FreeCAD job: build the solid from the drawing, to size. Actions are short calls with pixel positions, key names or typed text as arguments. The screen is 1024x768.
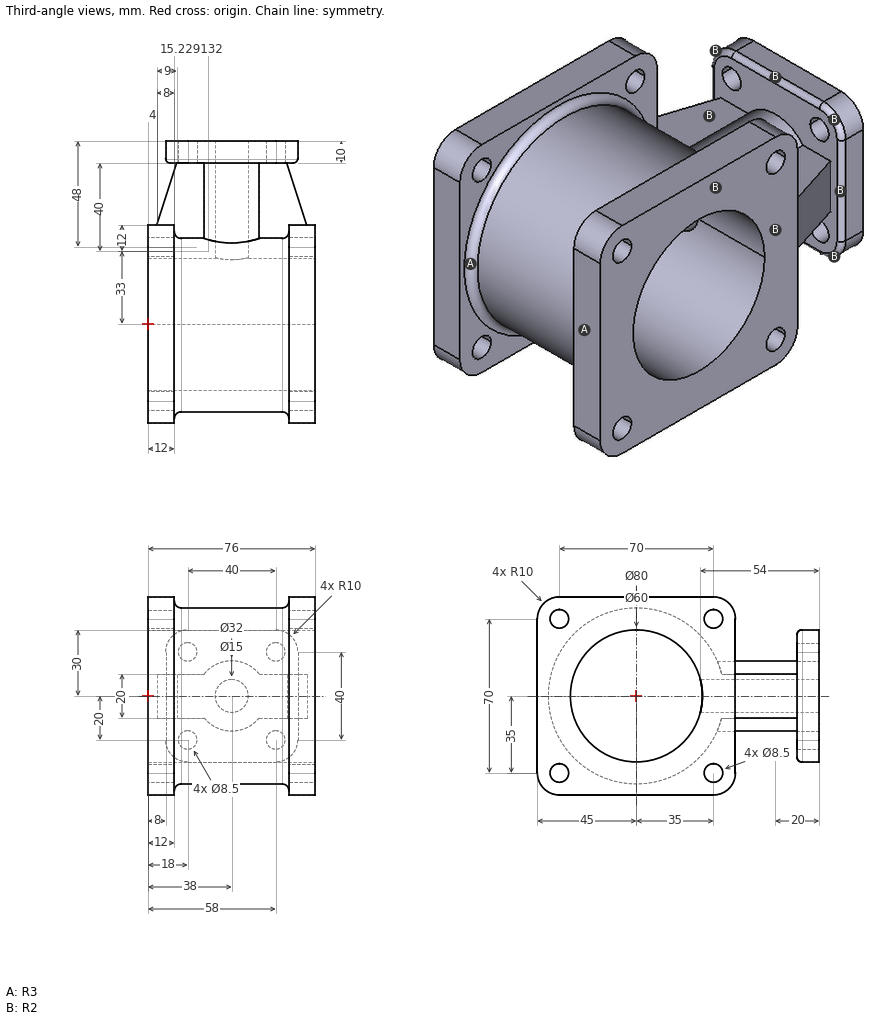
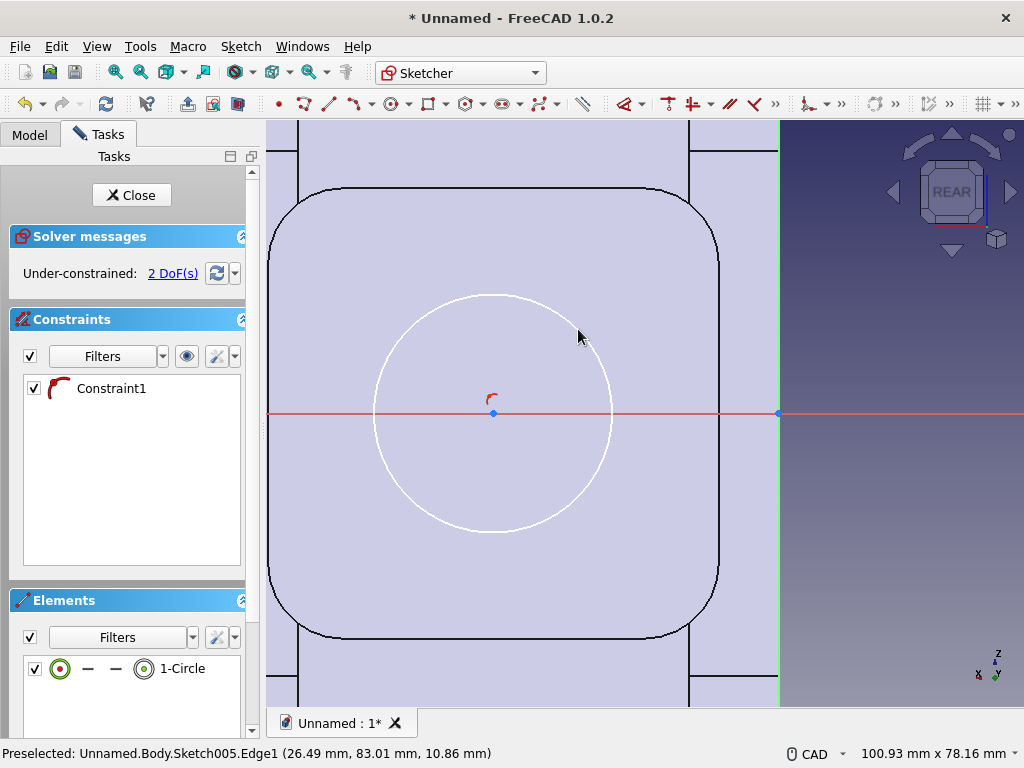
click(624, 104)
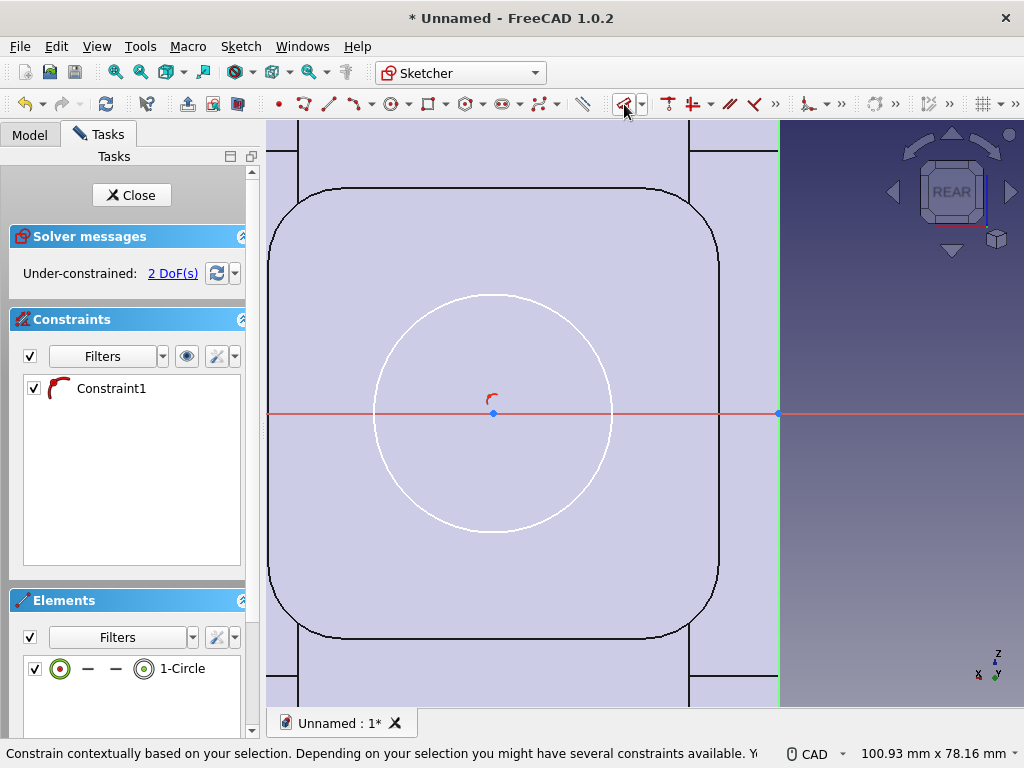
click(577, 329)
click(600, 306)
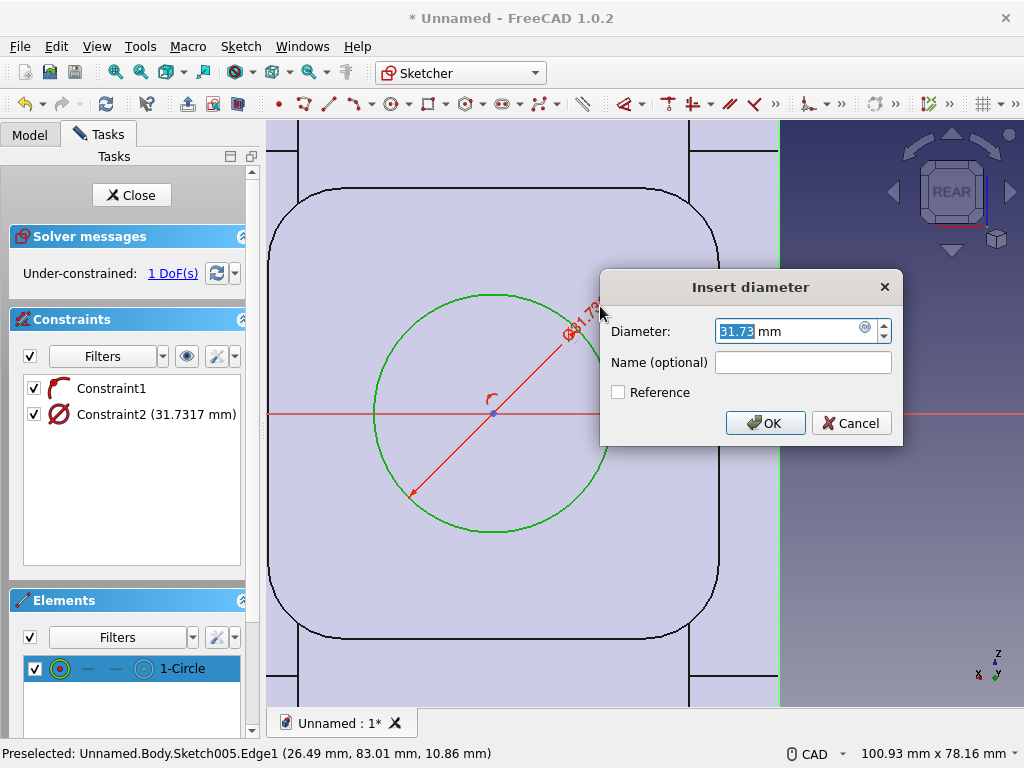
text(32)
key(Return)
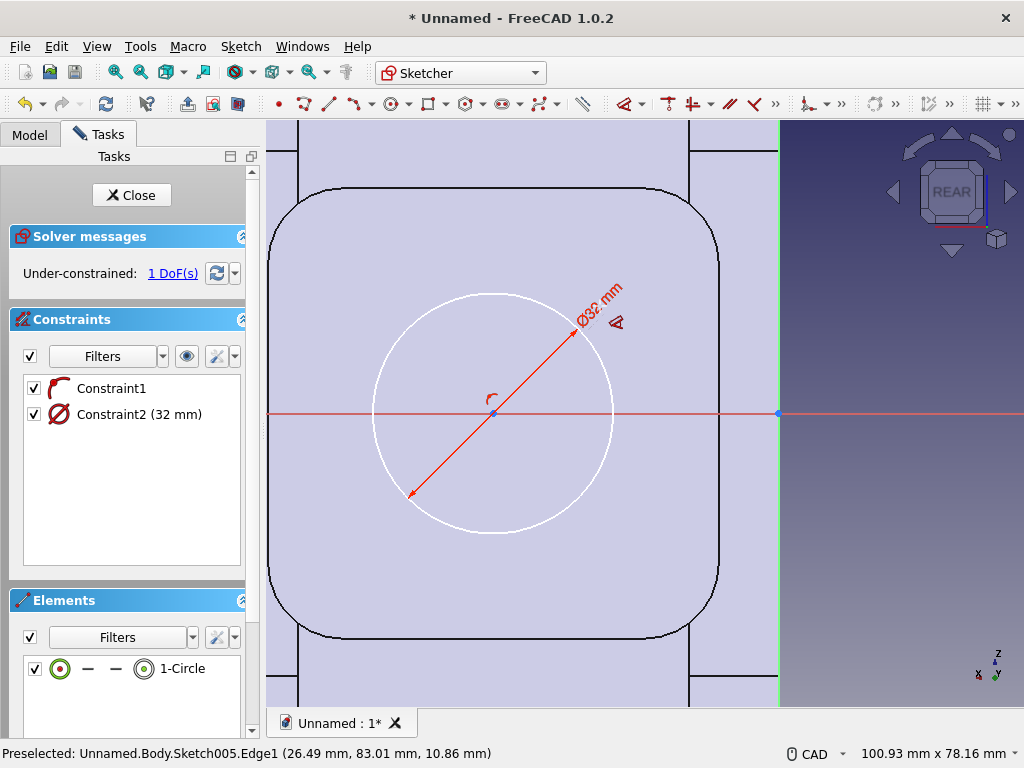
click(493, 413)
click(636, 447)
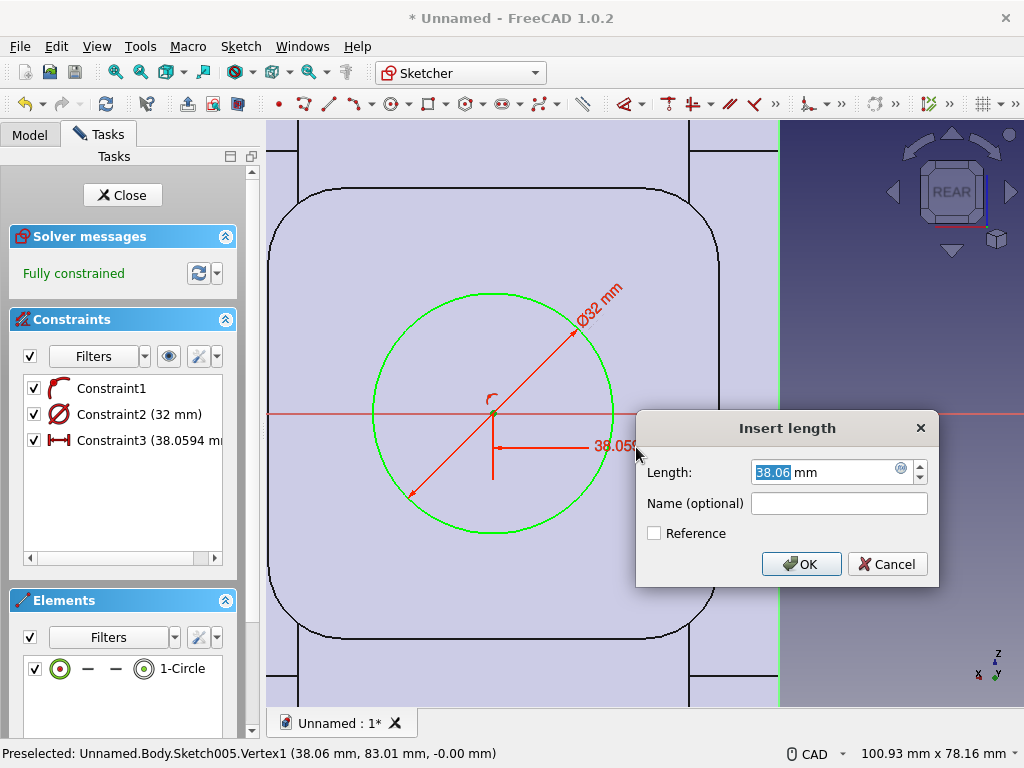
text(38)
key(Return)
key(Escape)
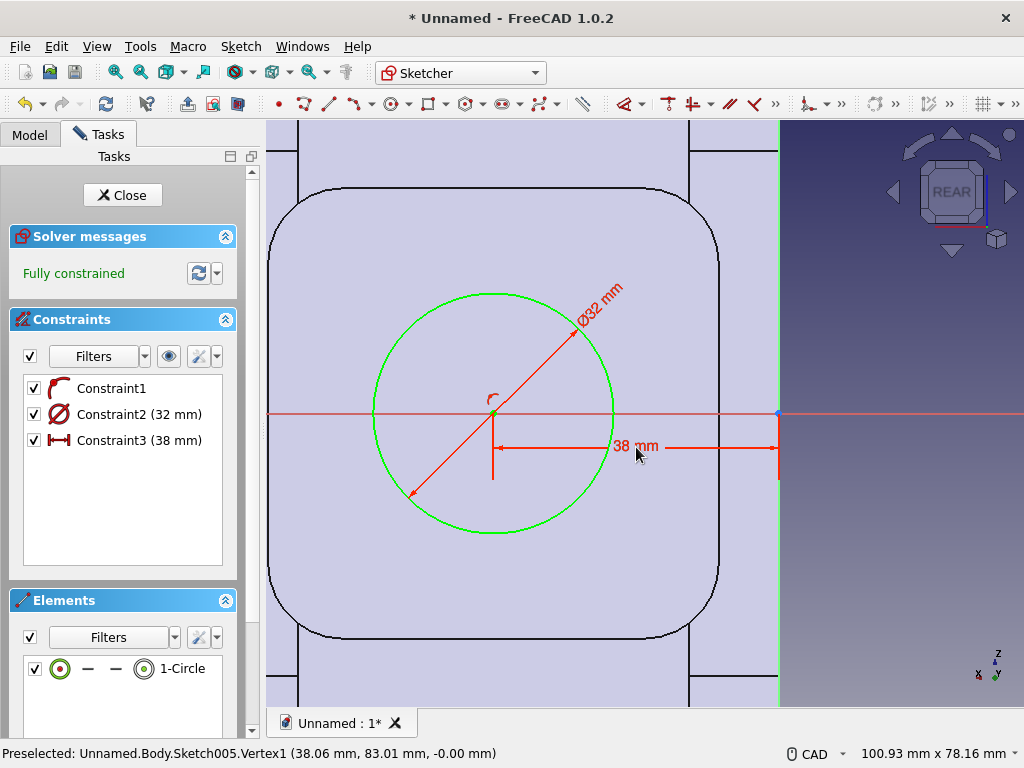
click(123, 195)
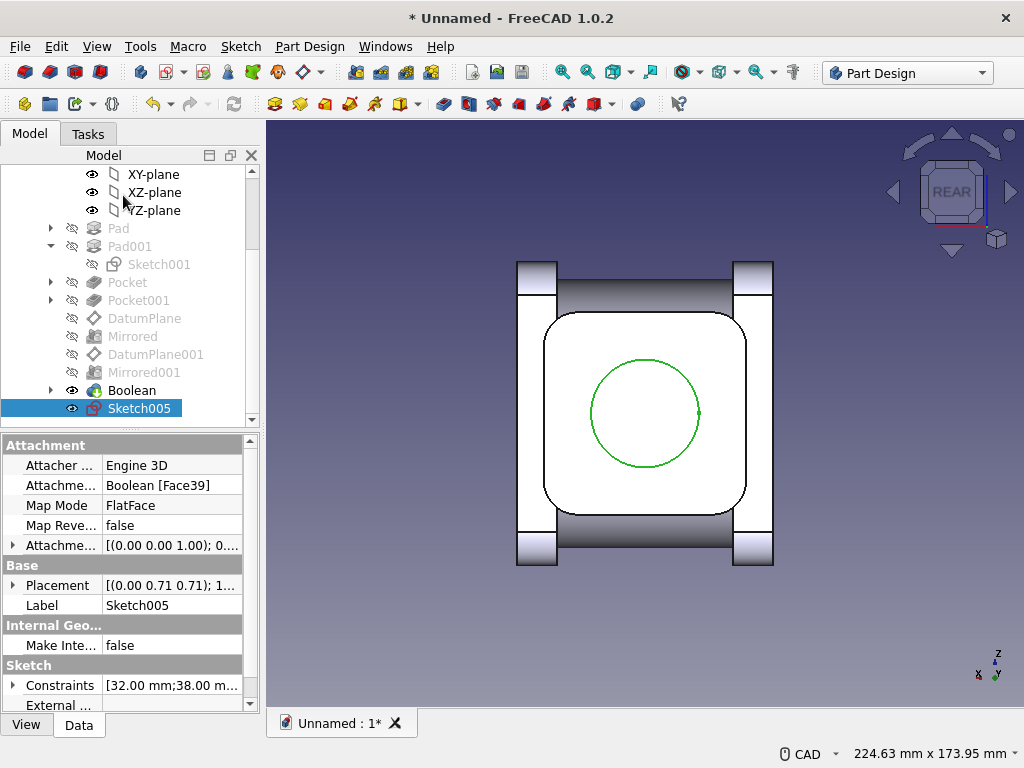
click(275, 104)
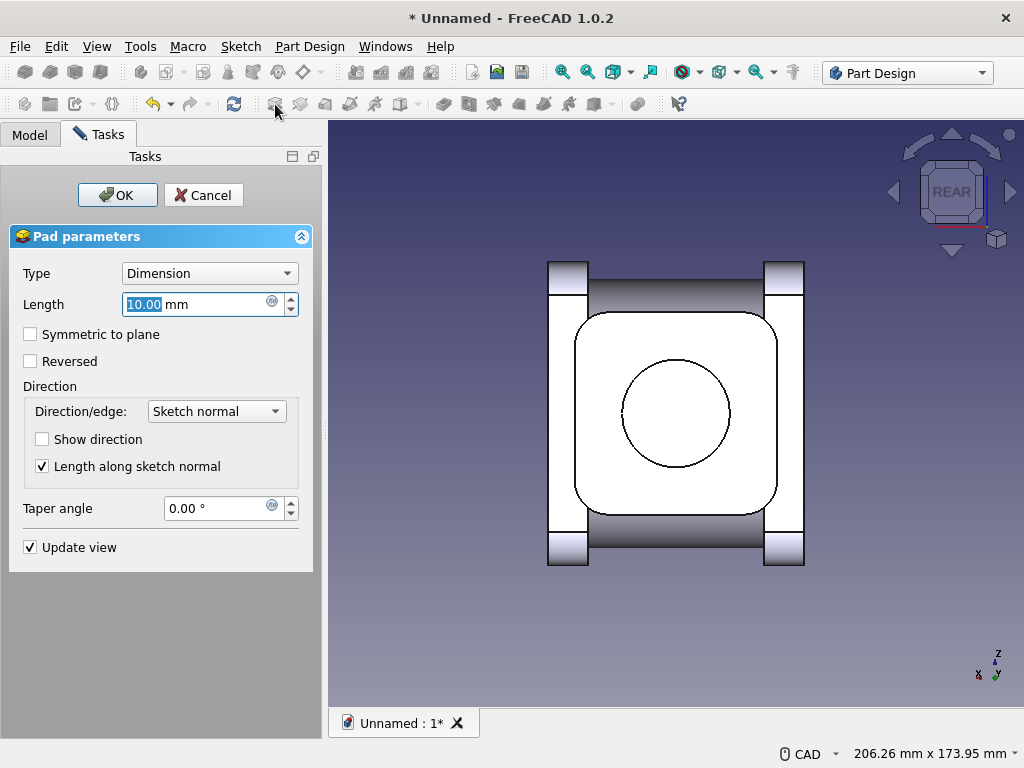
text(48)
key(Tab)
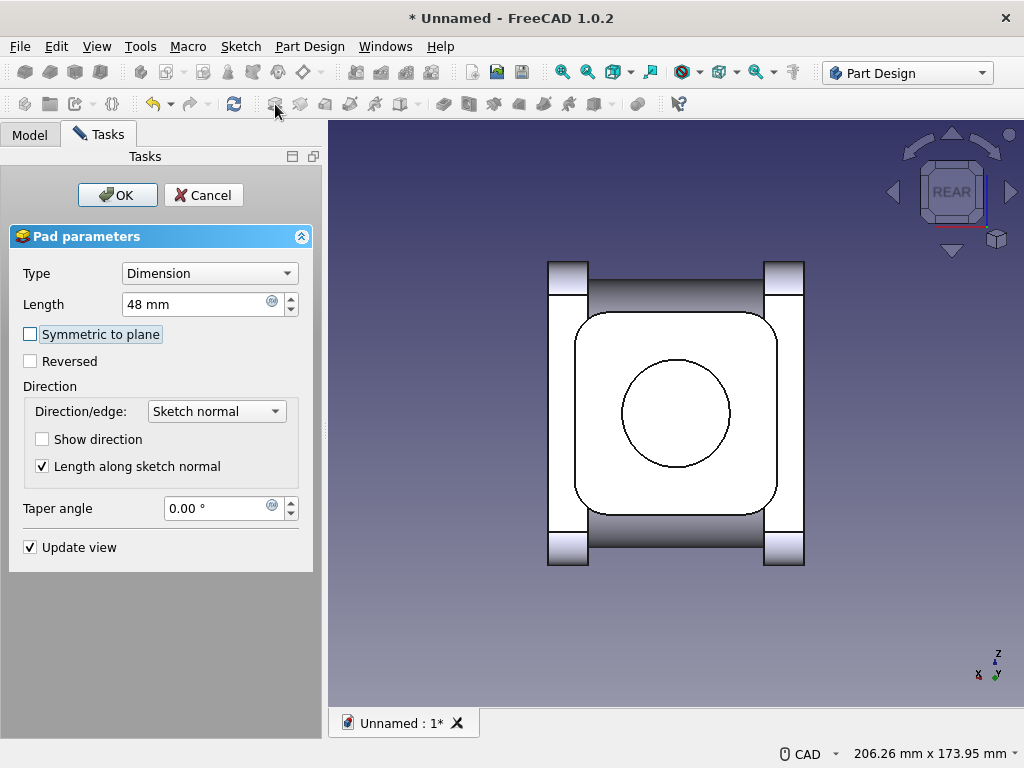
click(31, 361)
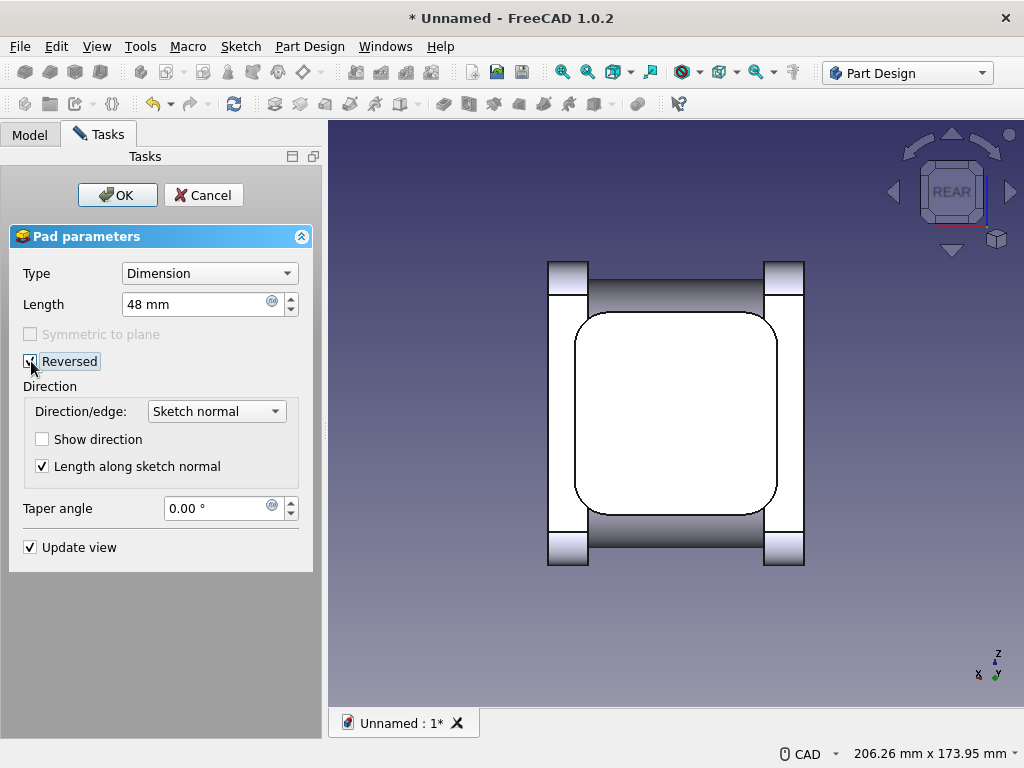
click(118, 195)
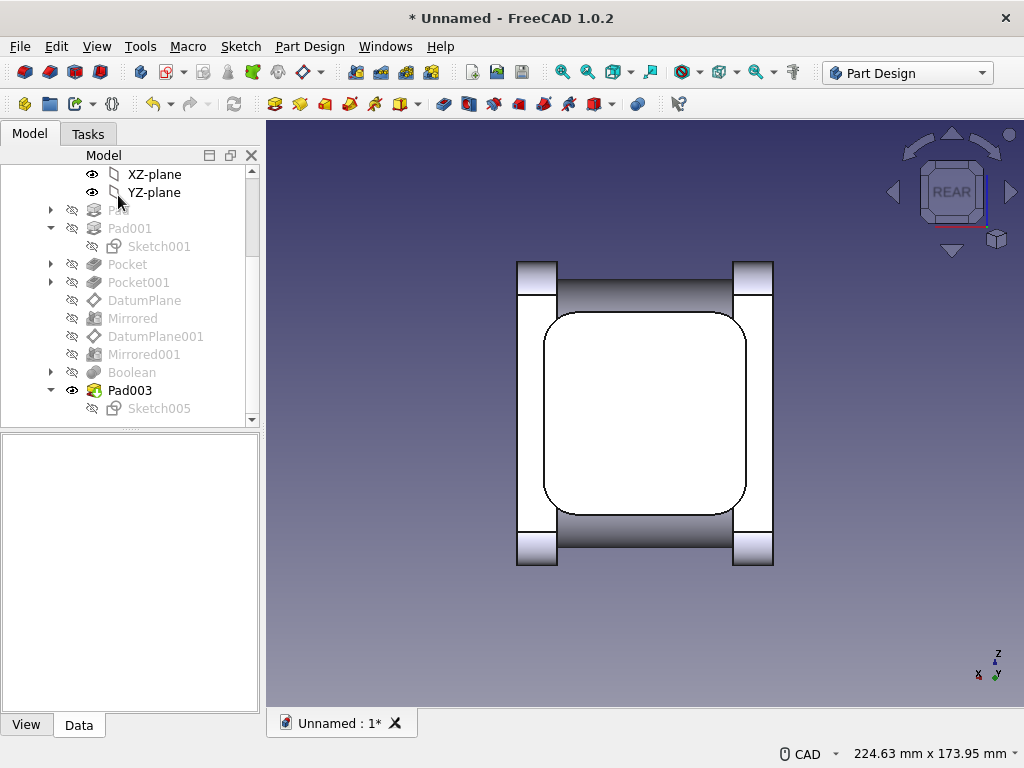
click(166, 72)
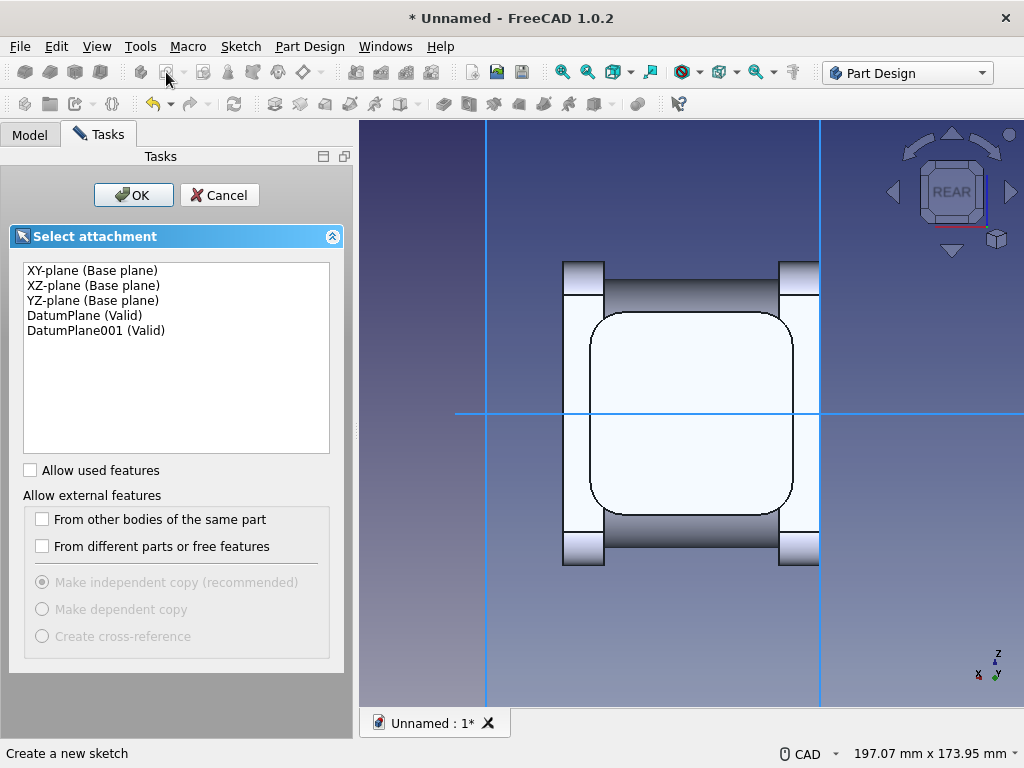
click(84, 270)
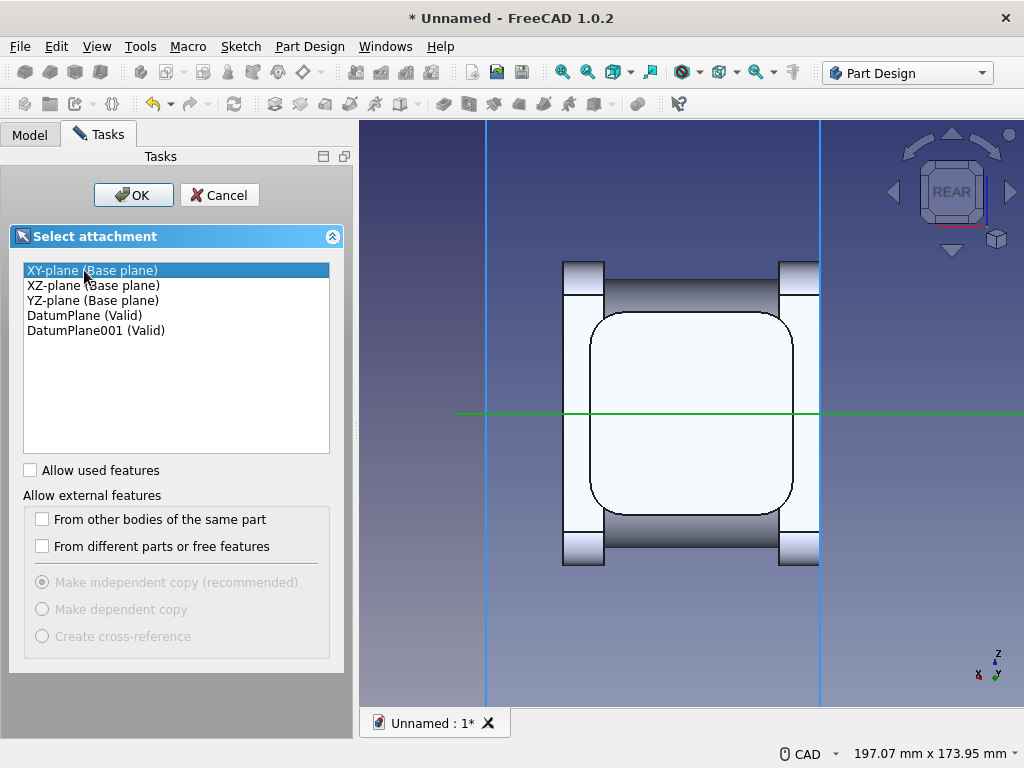
click(134, 195)